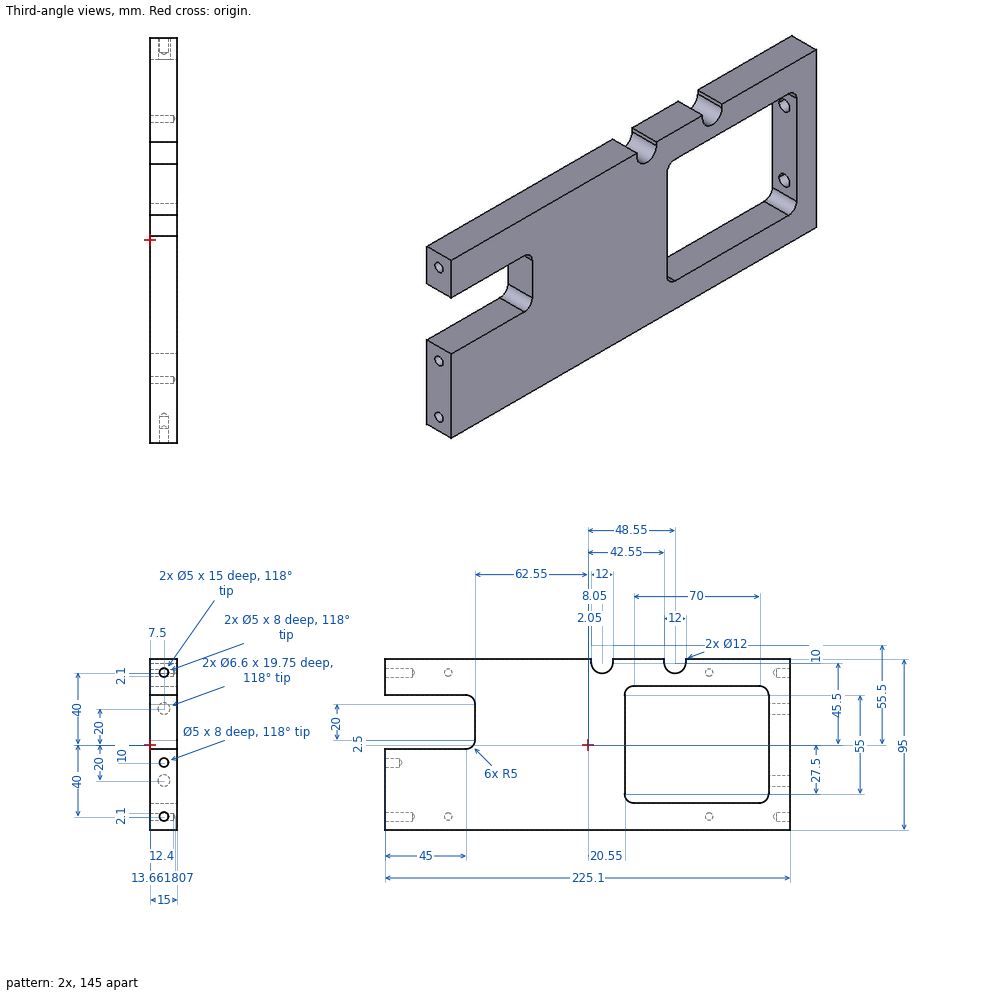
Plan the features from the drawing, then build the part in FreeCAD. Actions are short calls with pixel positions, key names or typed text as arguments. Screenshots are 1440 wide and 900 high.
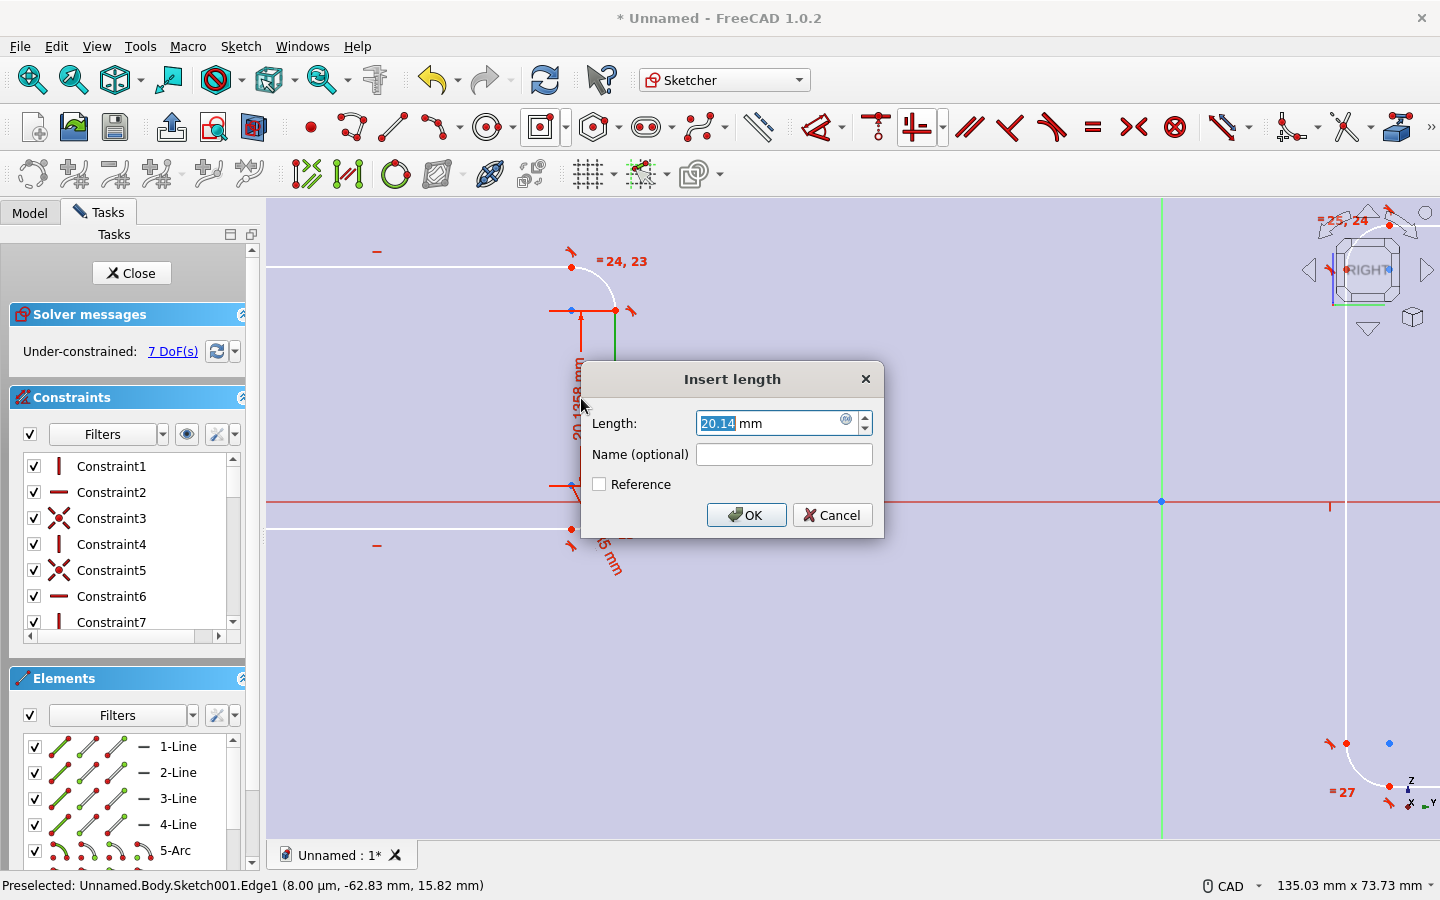
text(20)
key(Return)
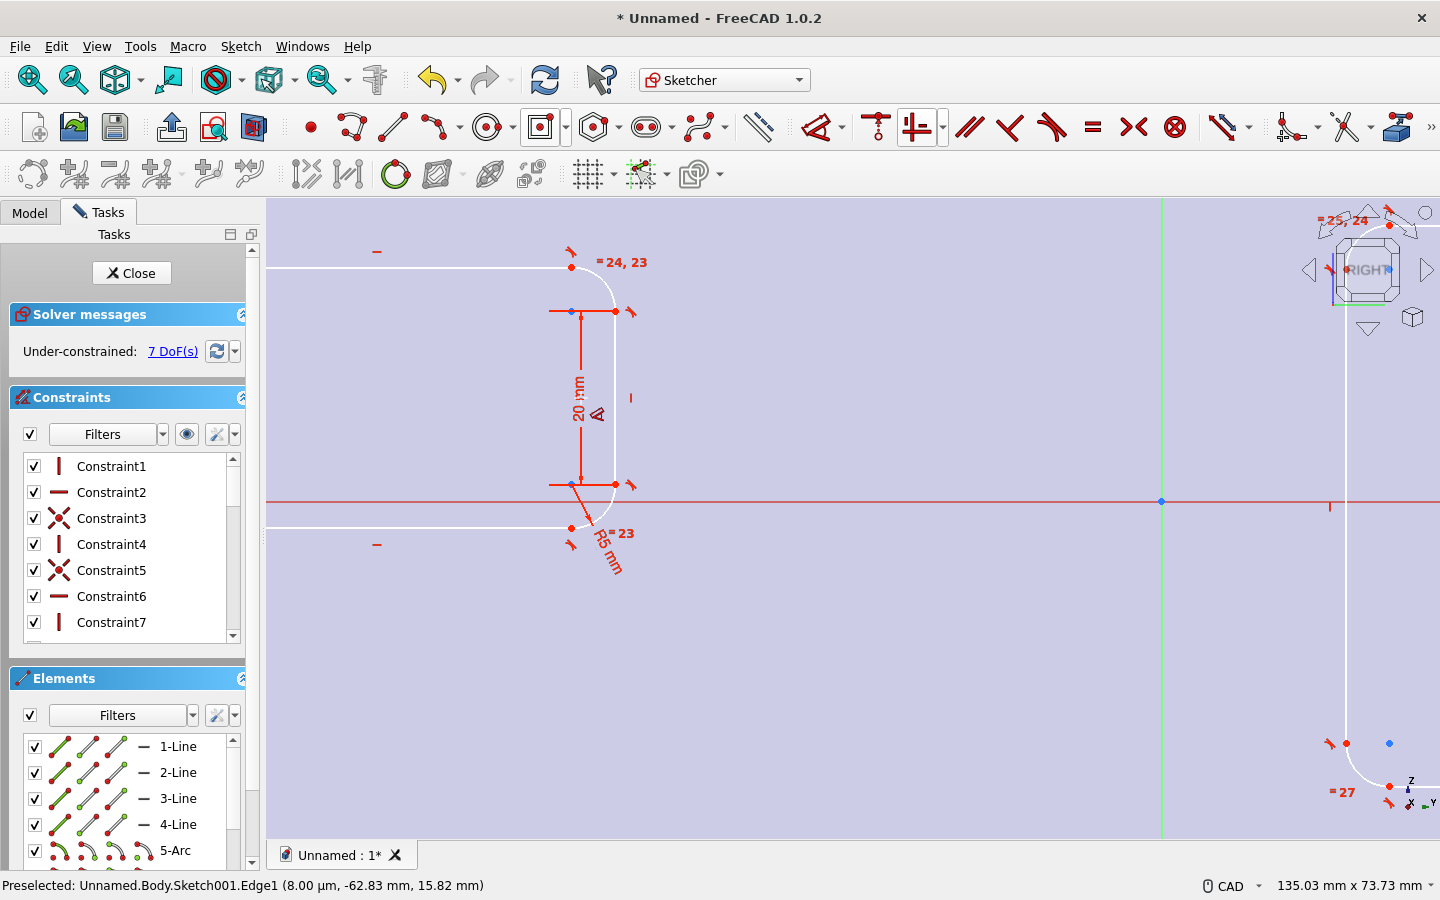
click(455, 528)
click(433, 562)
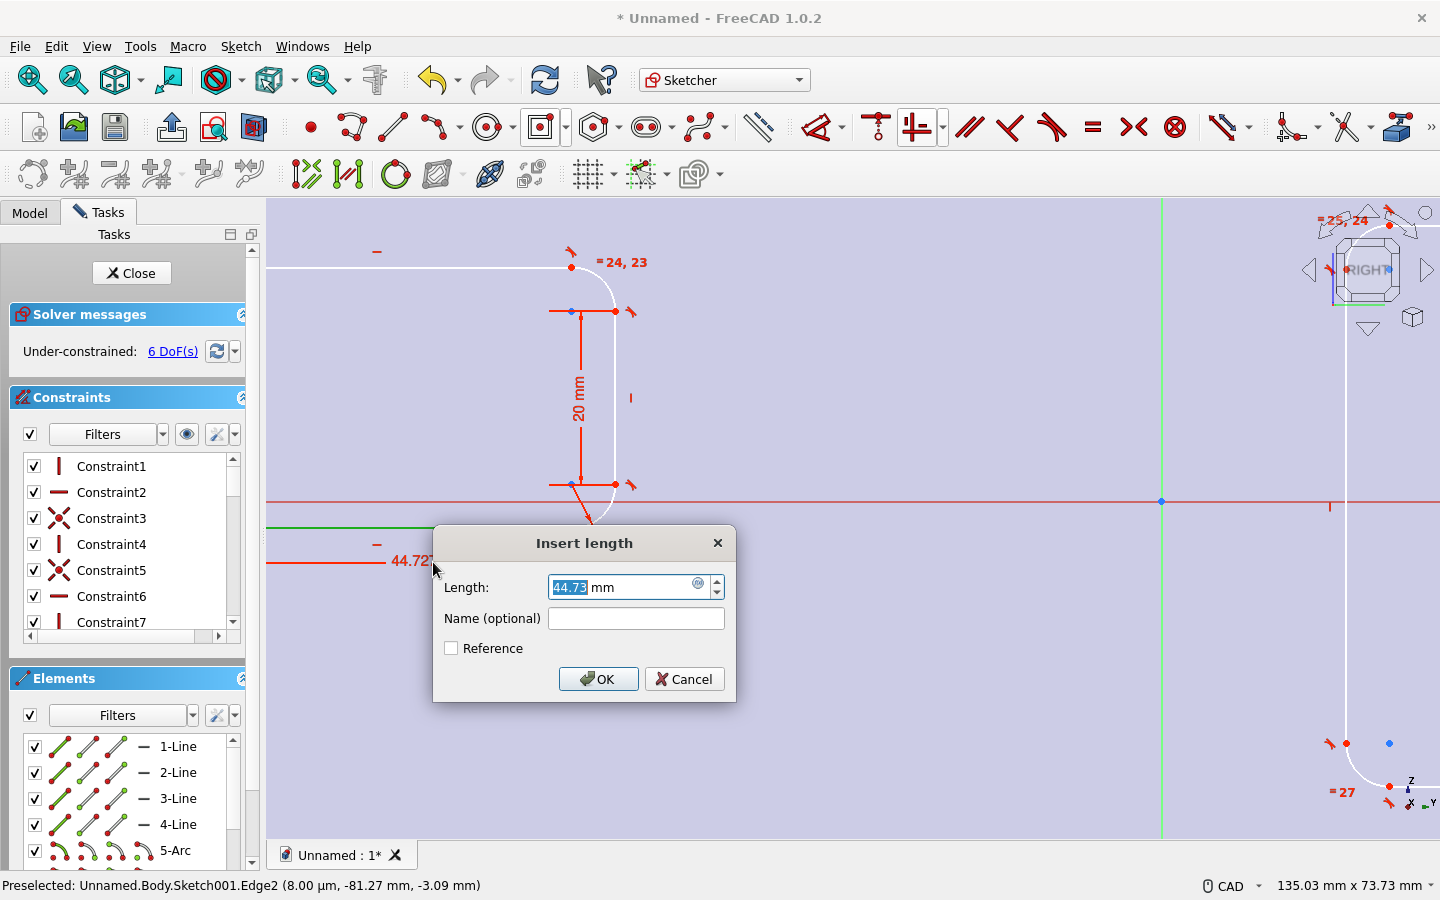
text(45)
key(Return)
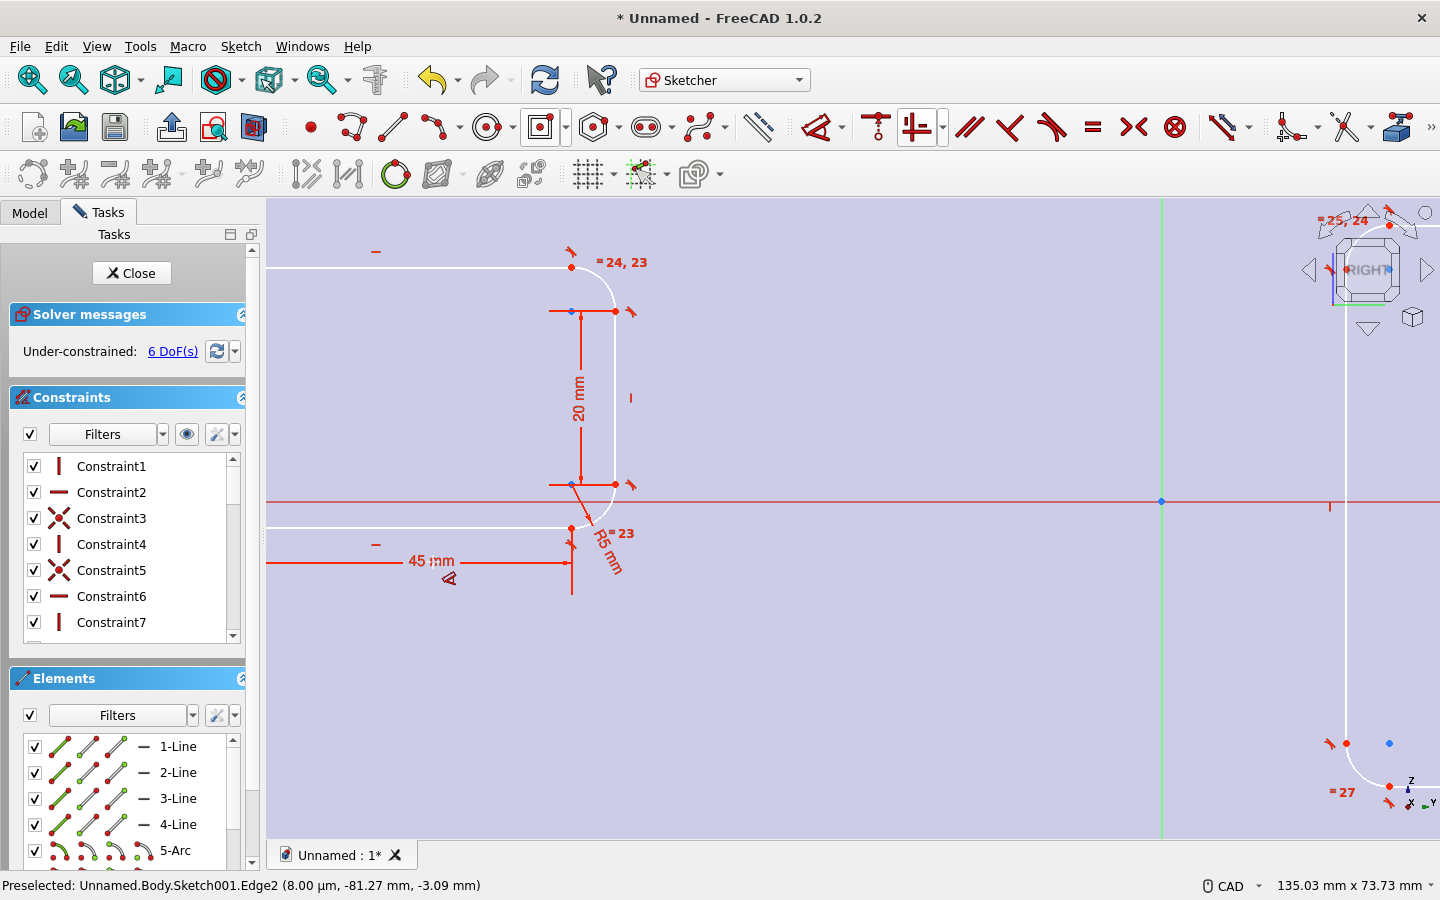
scroll(595, 528, down, 5)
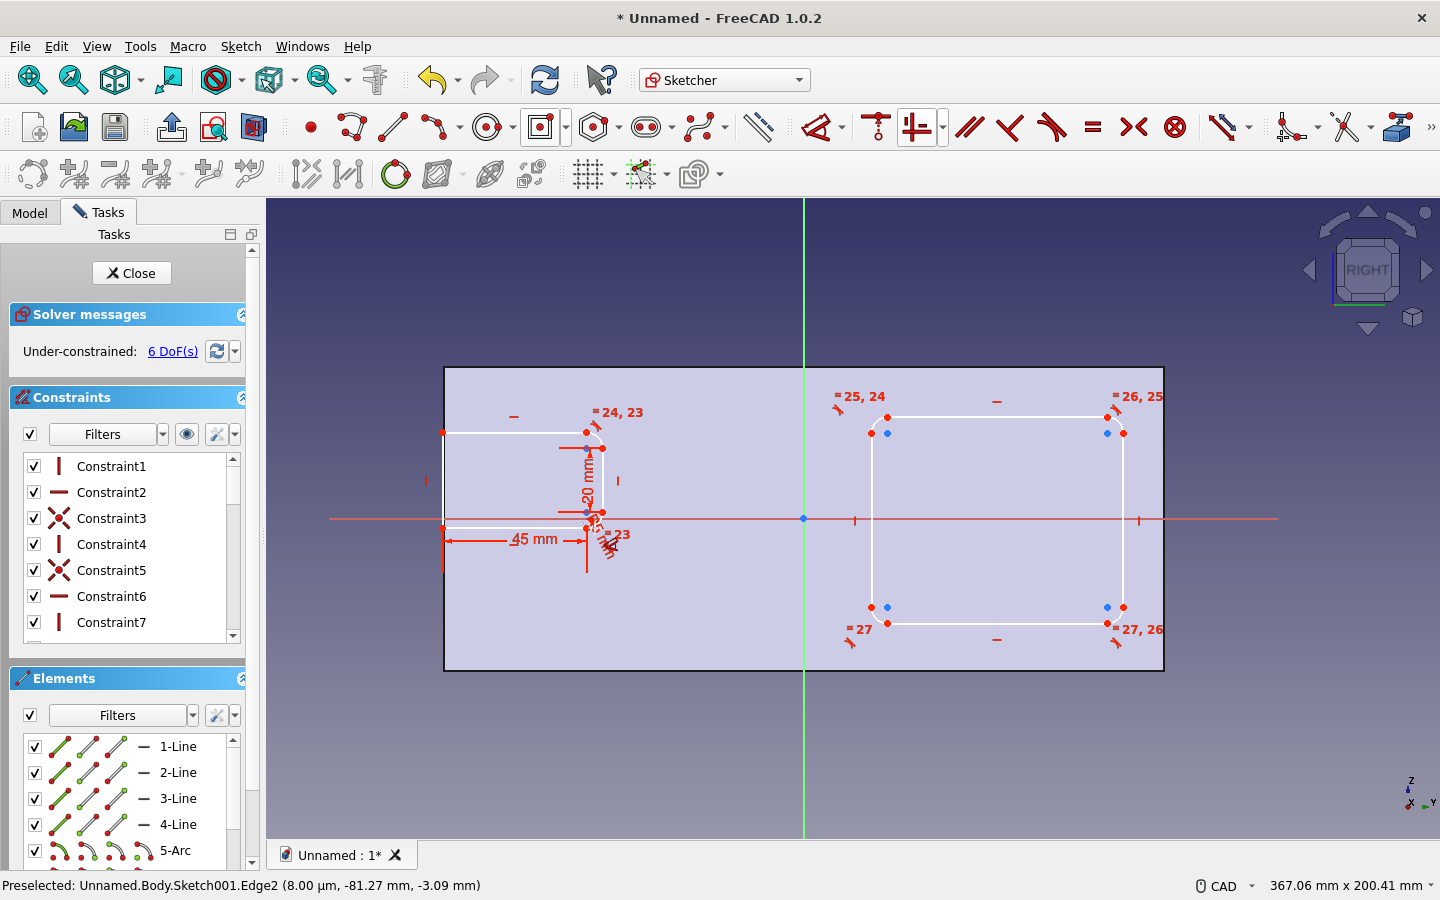
click(872, 555)
click(906, 480)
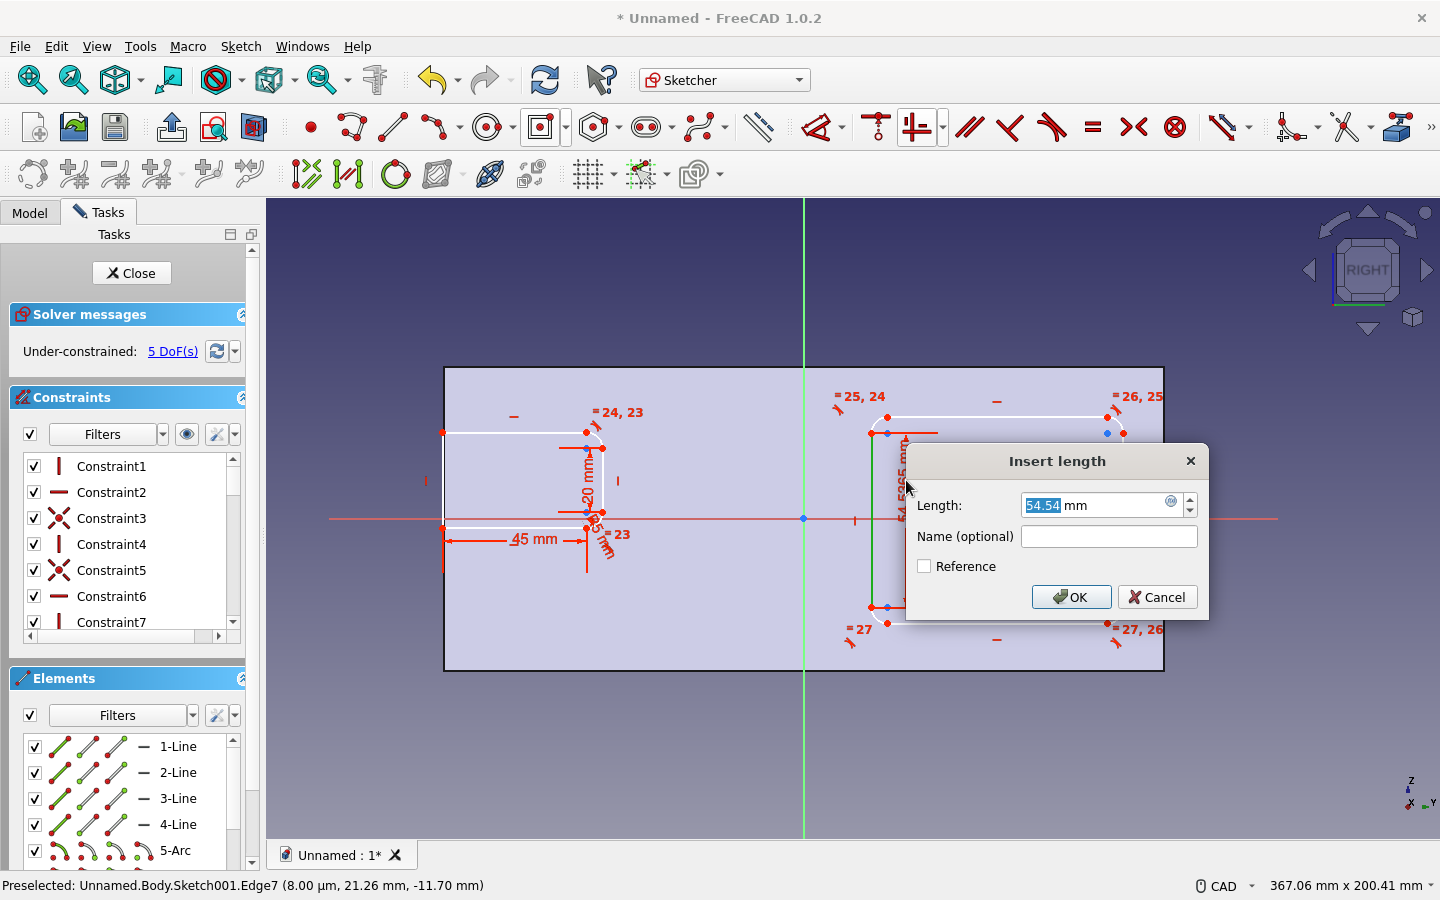
text(55)
key(Return)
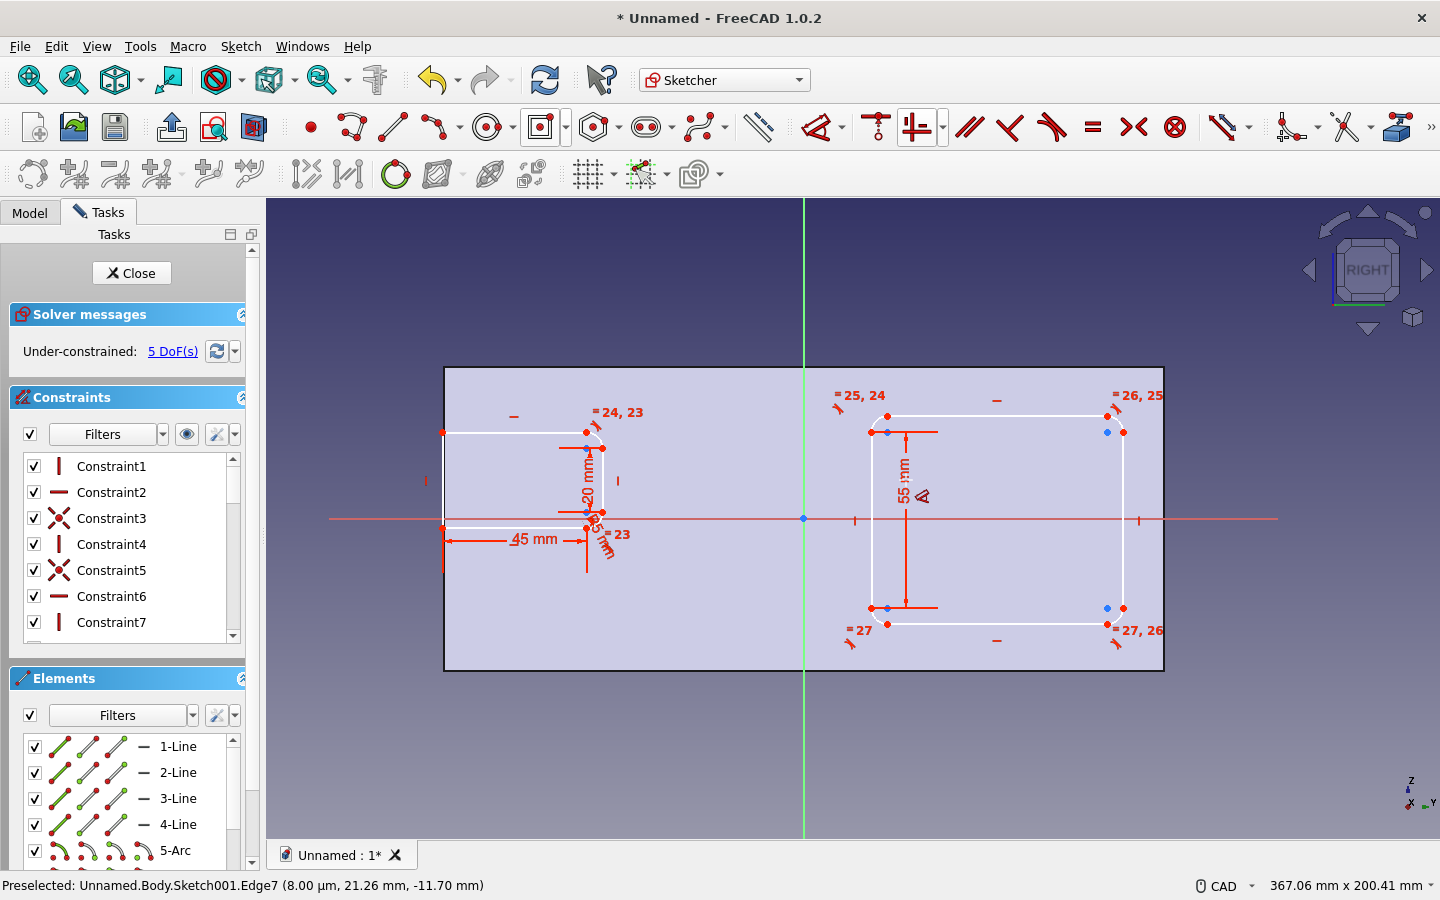
click(953, 416)
click(997, 382)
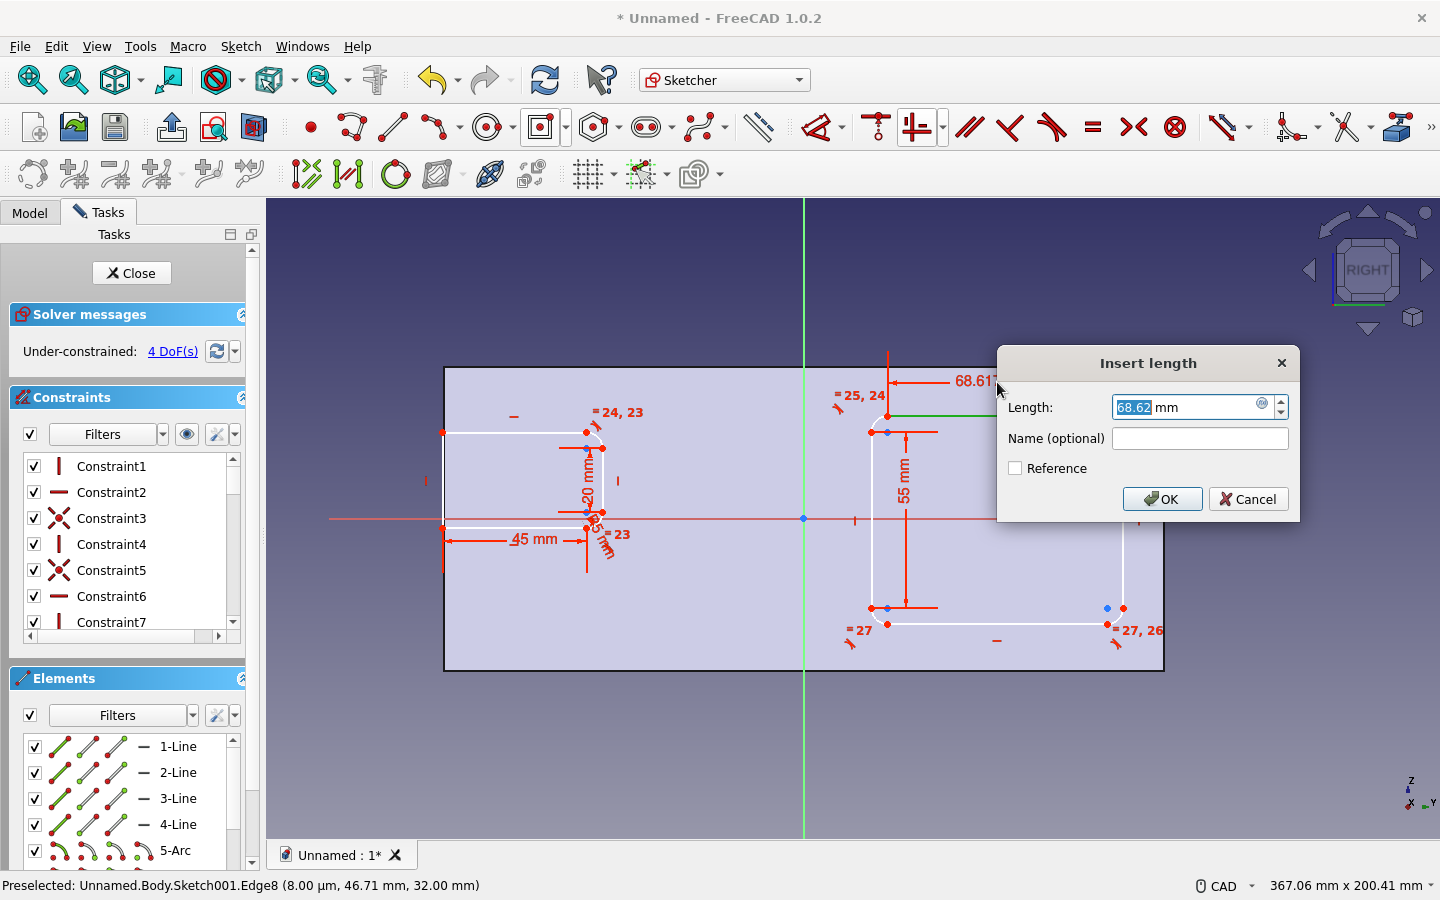
text(70)
key(Return)